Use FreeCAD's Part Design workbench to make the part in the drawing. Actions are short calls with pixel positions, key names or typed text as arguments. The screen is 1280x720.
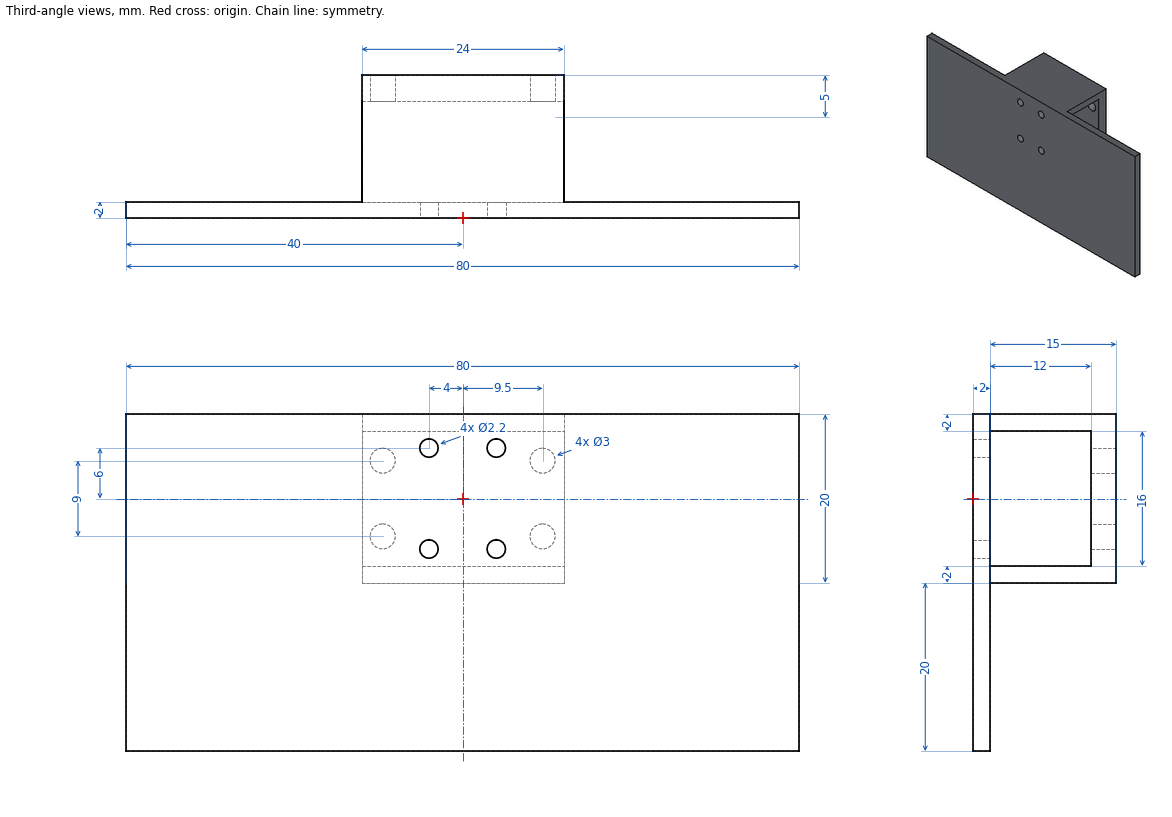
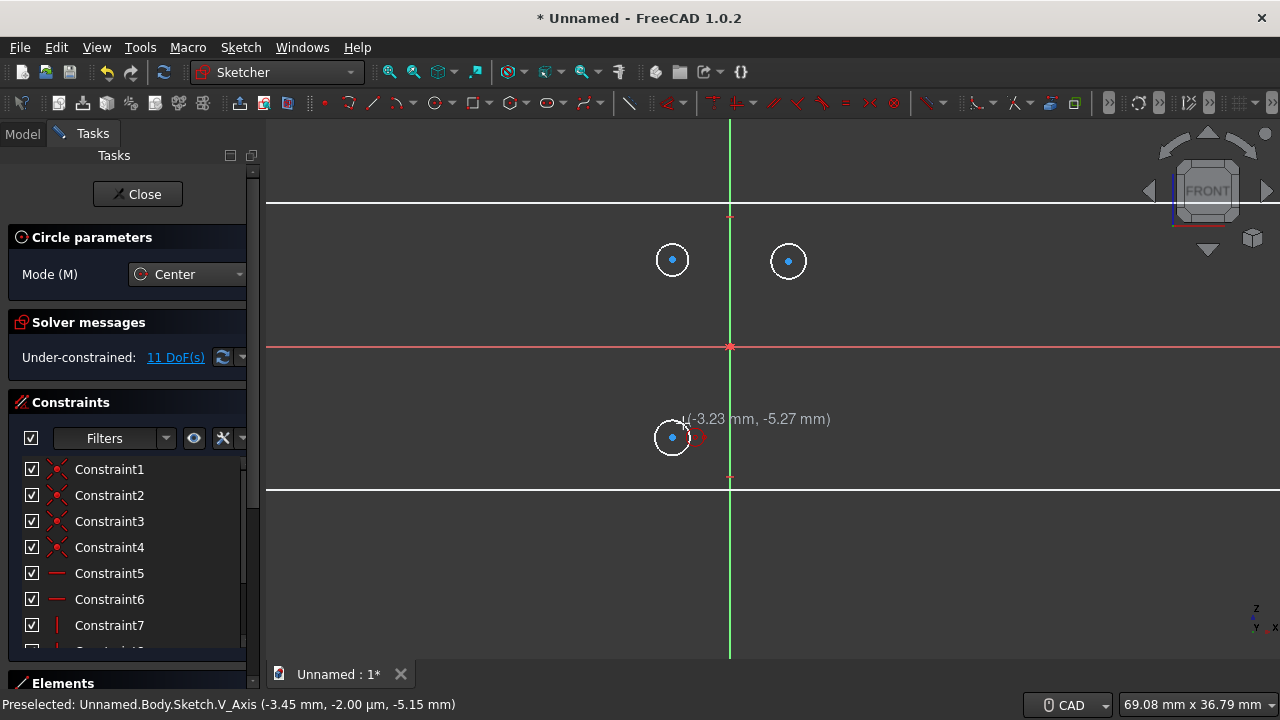
scroll(789, 435, up, 2)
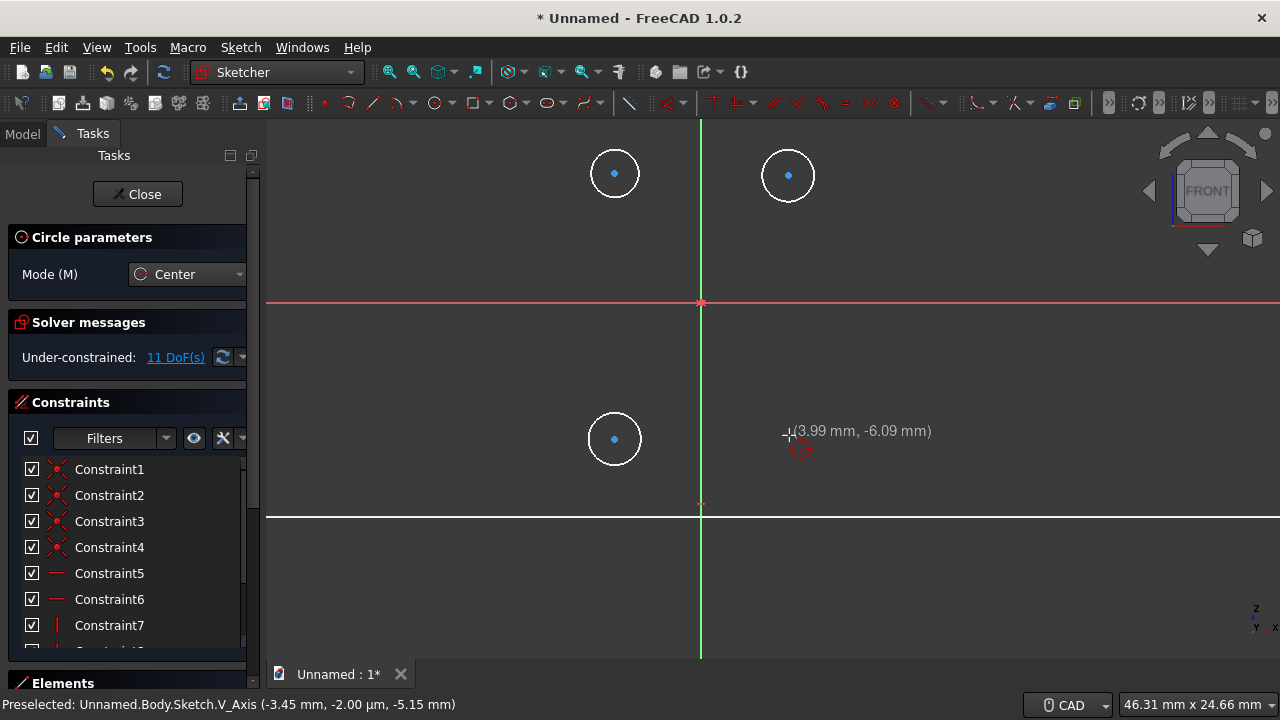
scroll(706, 426, down, 6)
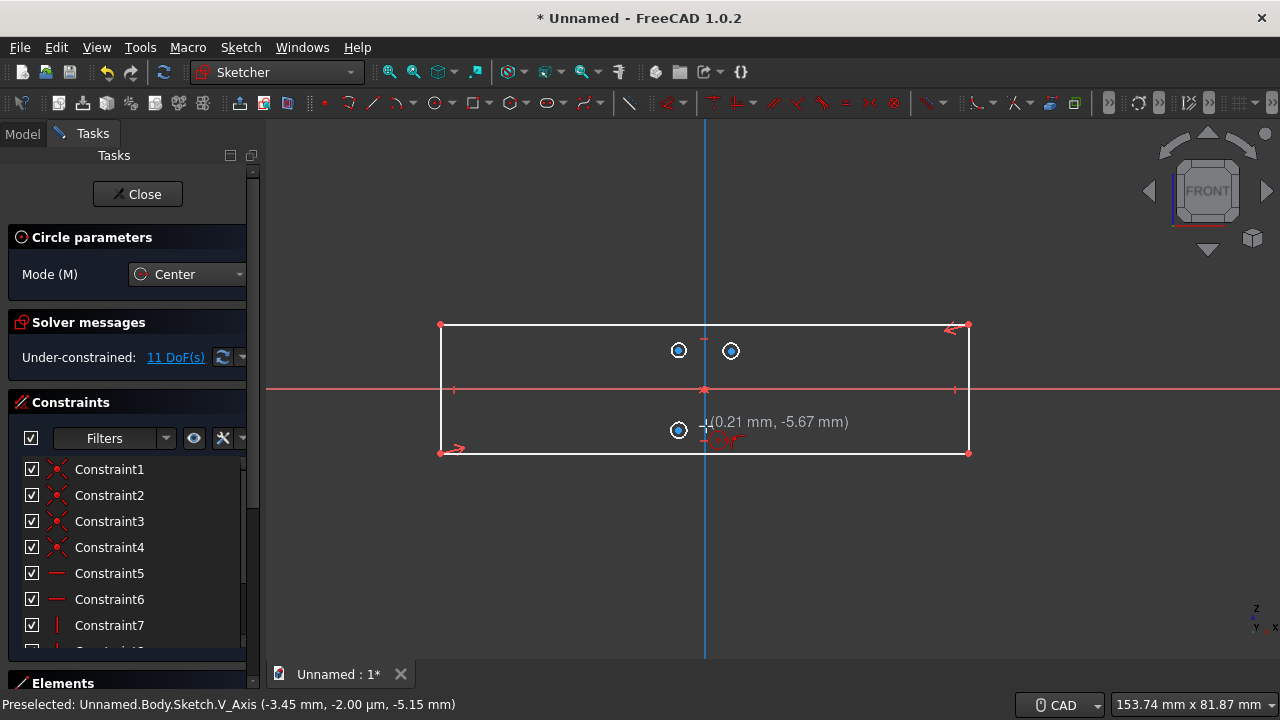
click(731, 429)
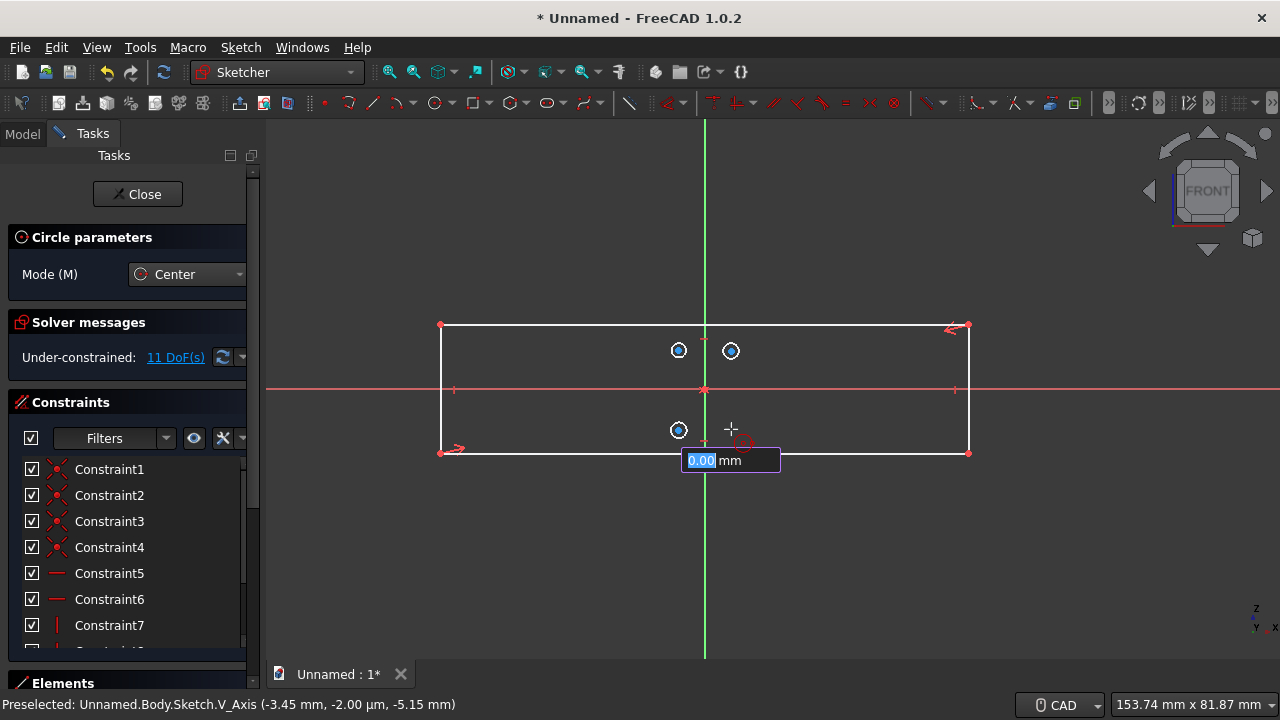
scroll(736, 424, up, 4)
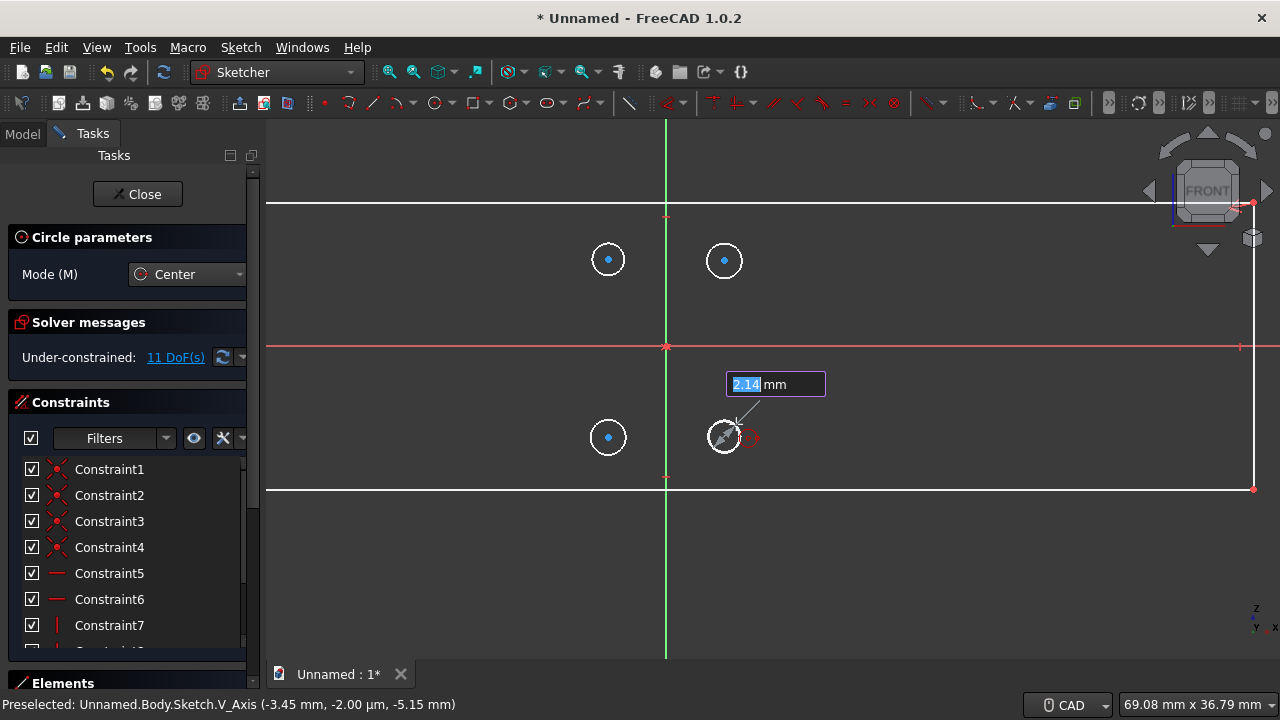
click(736, 423)
key(Escape)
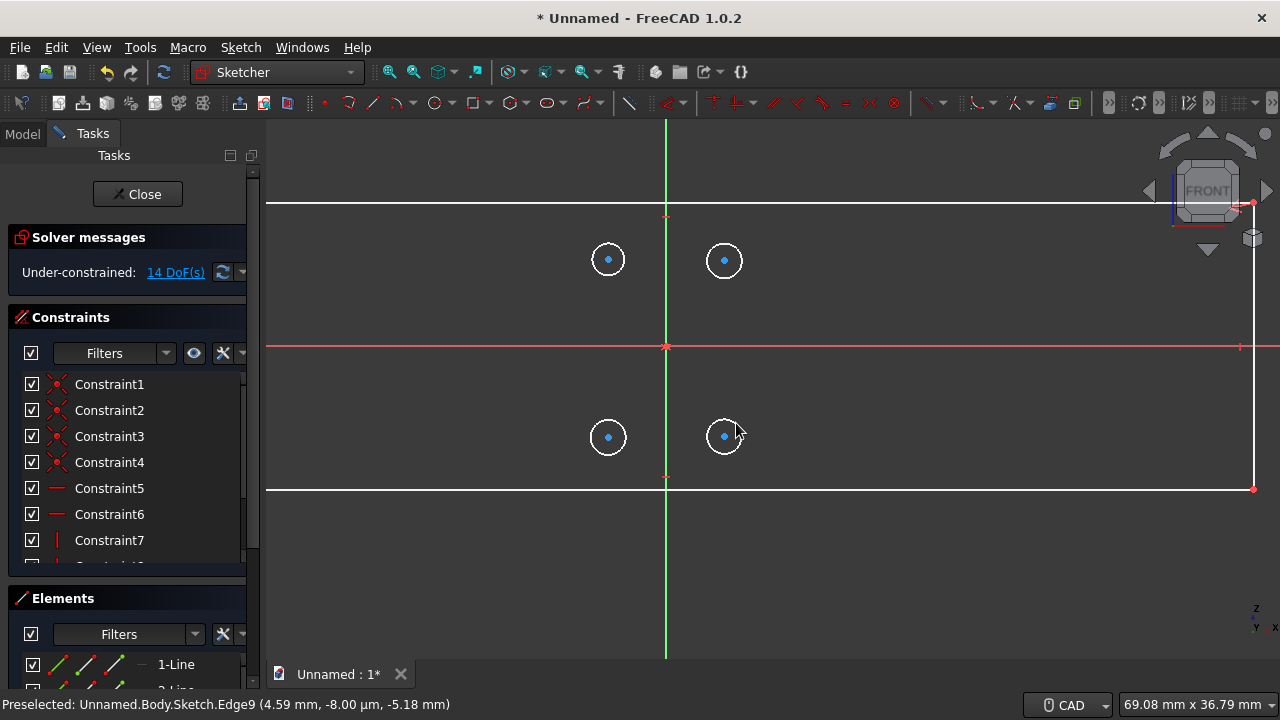
click(620, 248)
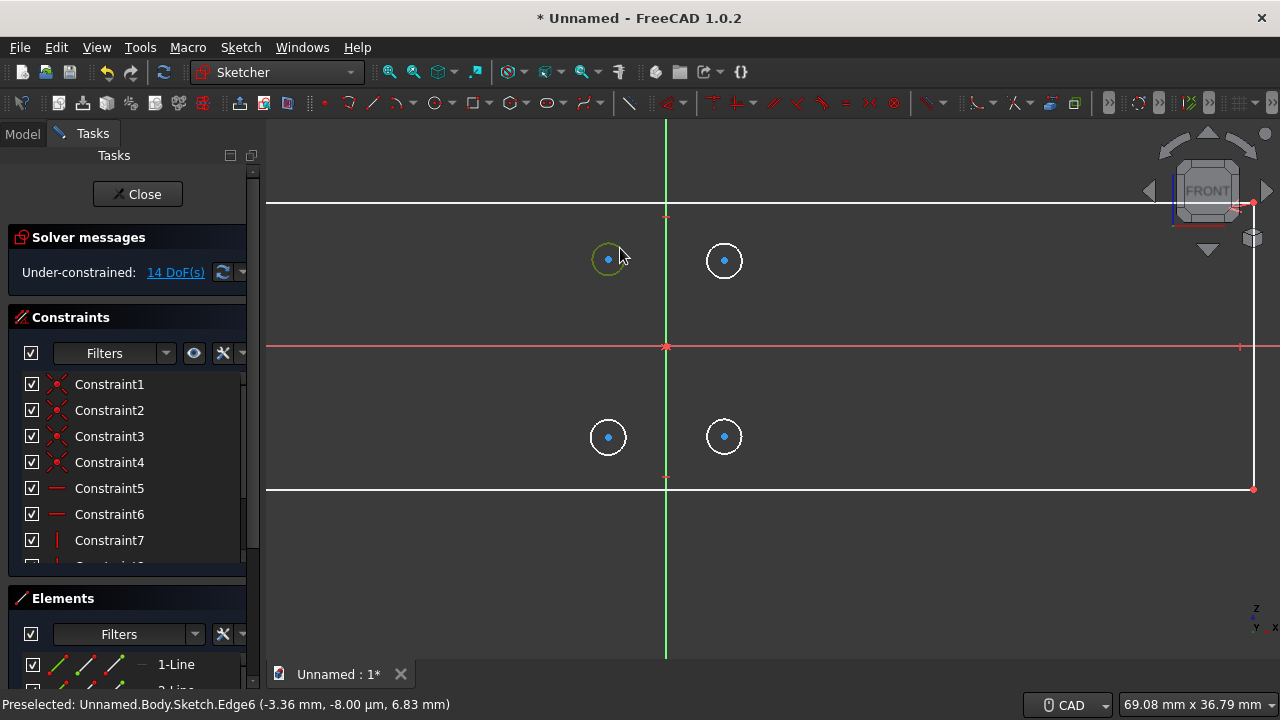
click(737, 249)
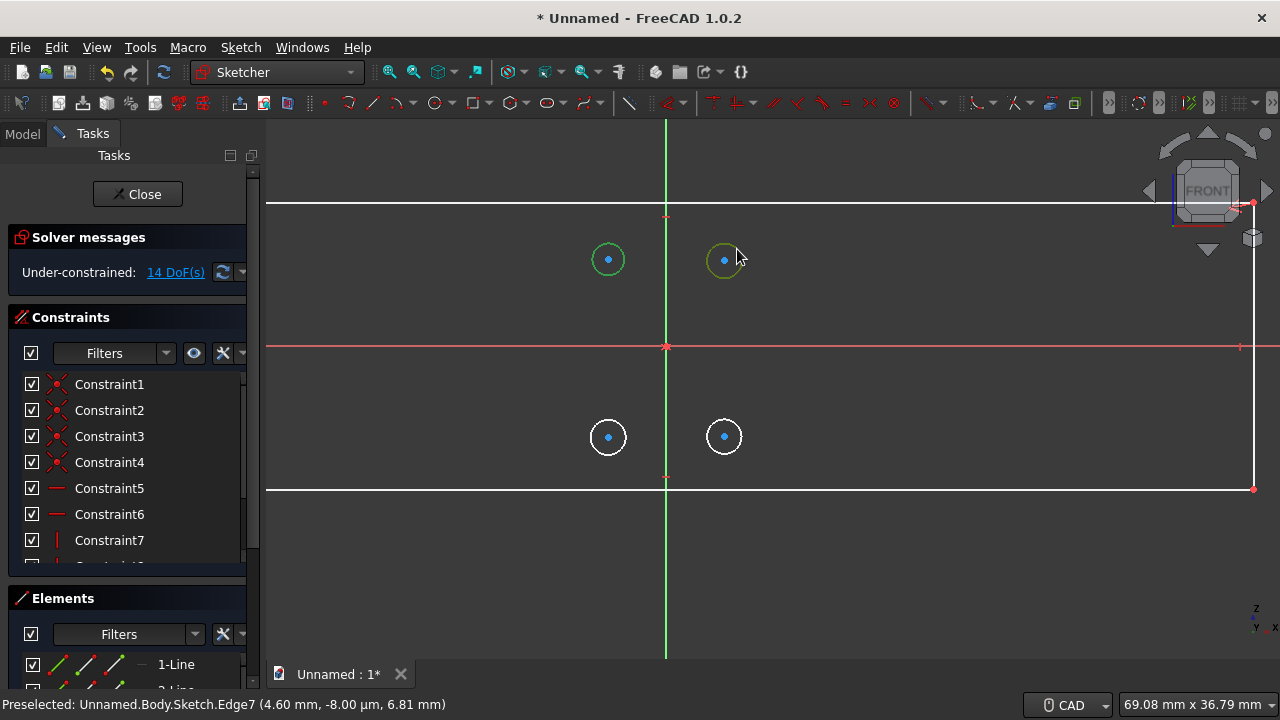
click(621, 425)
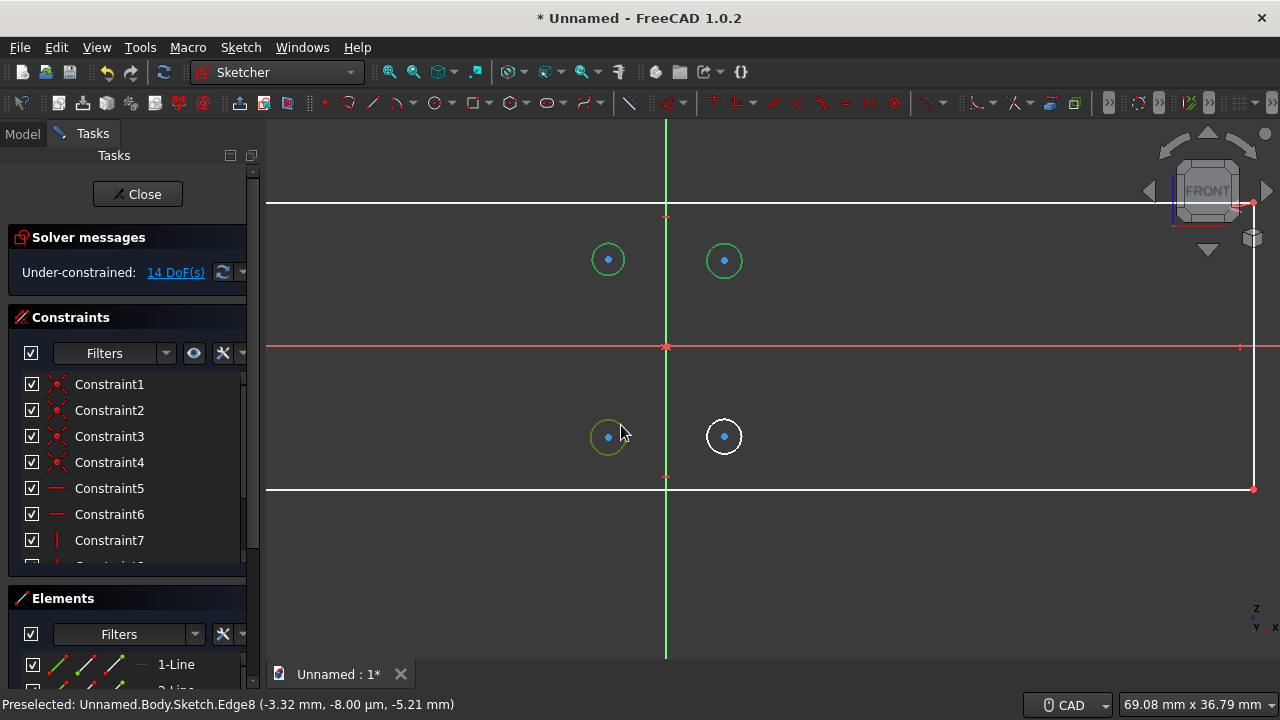
click(736, 424)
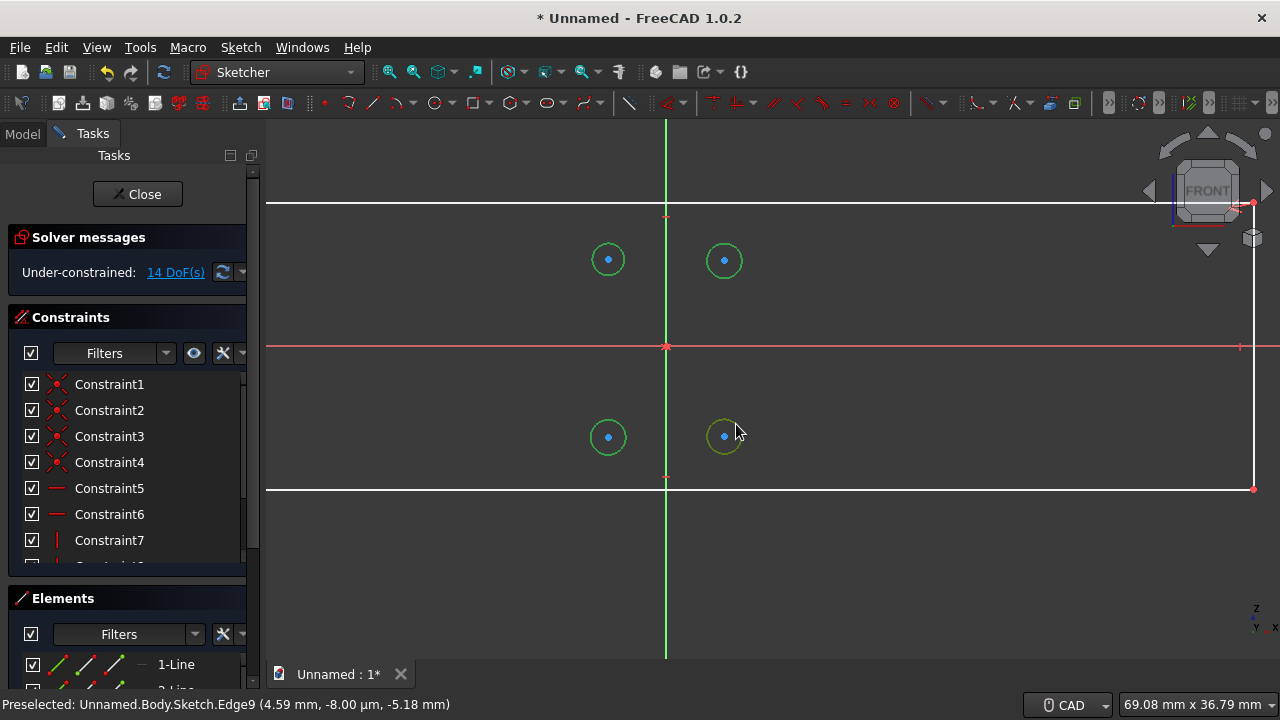
click(846, 104)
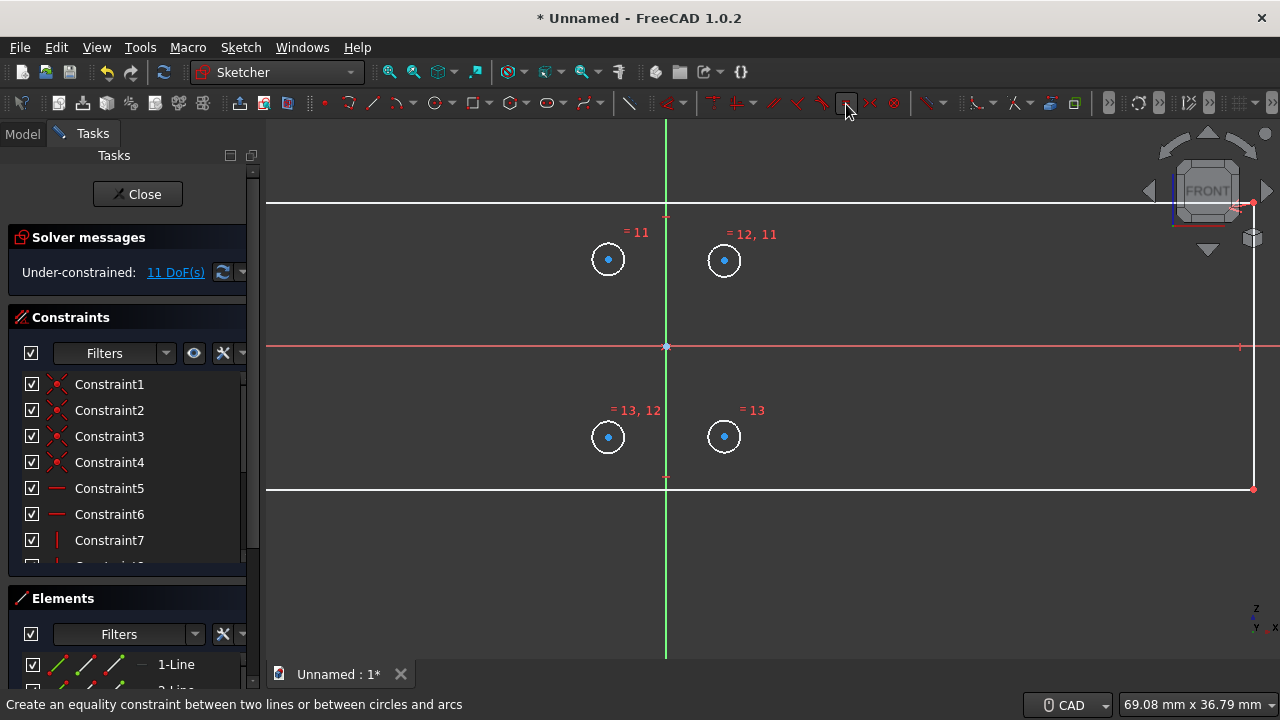
click(608, 259)